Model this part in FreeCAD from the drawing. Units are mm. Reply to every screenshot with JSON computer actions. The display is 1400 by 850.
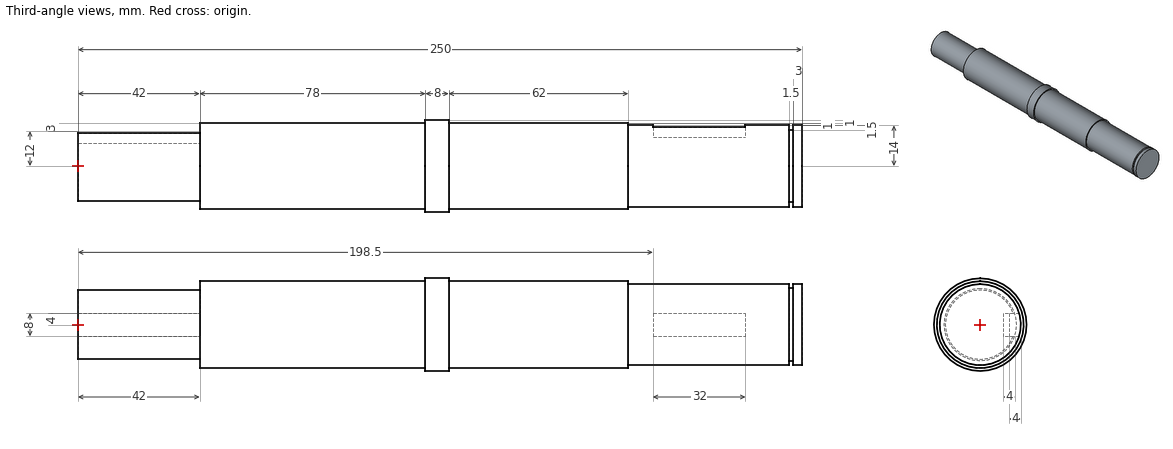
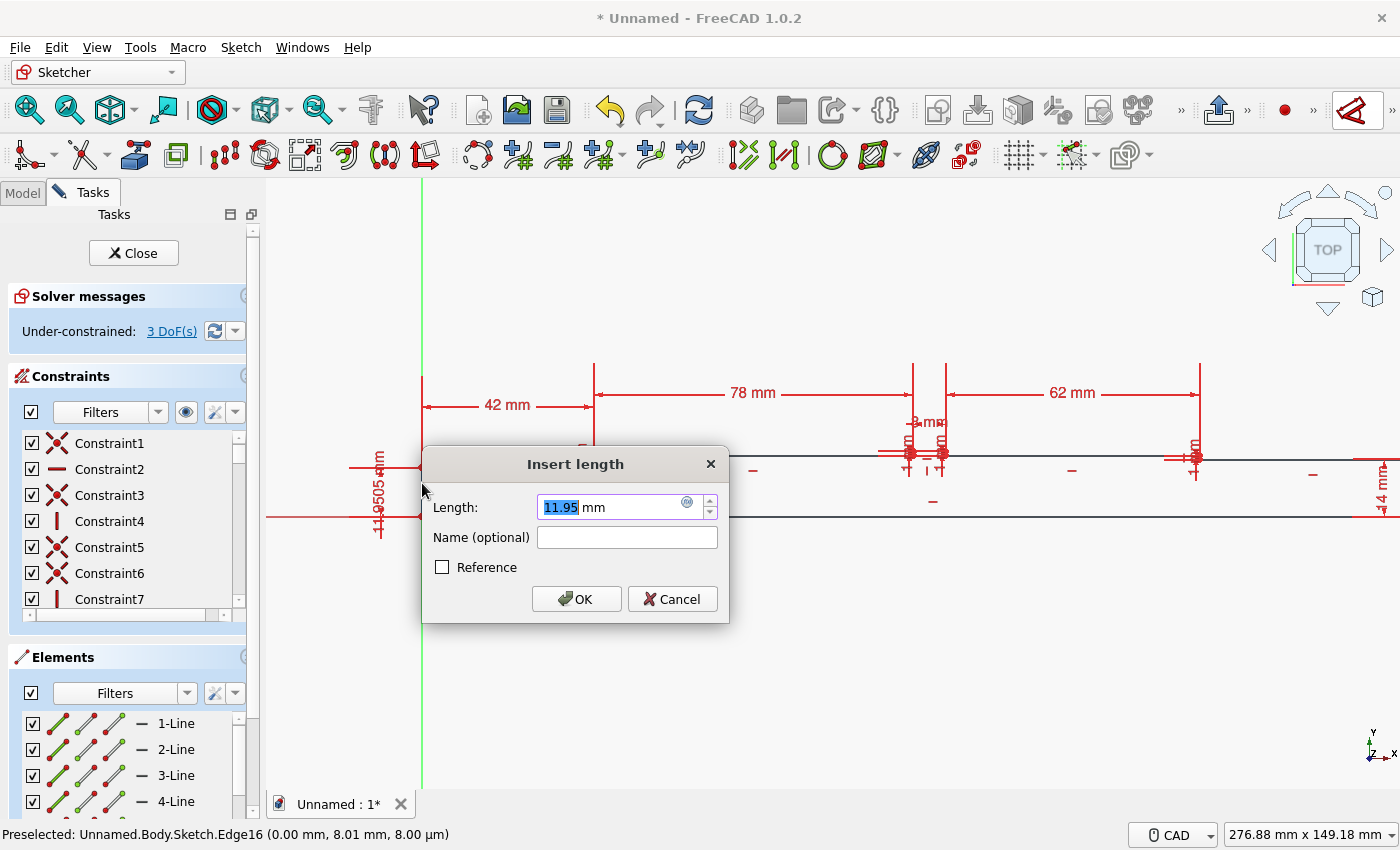
{"action": "type", "text": "12"}
{"action": "key", "text": "Return"}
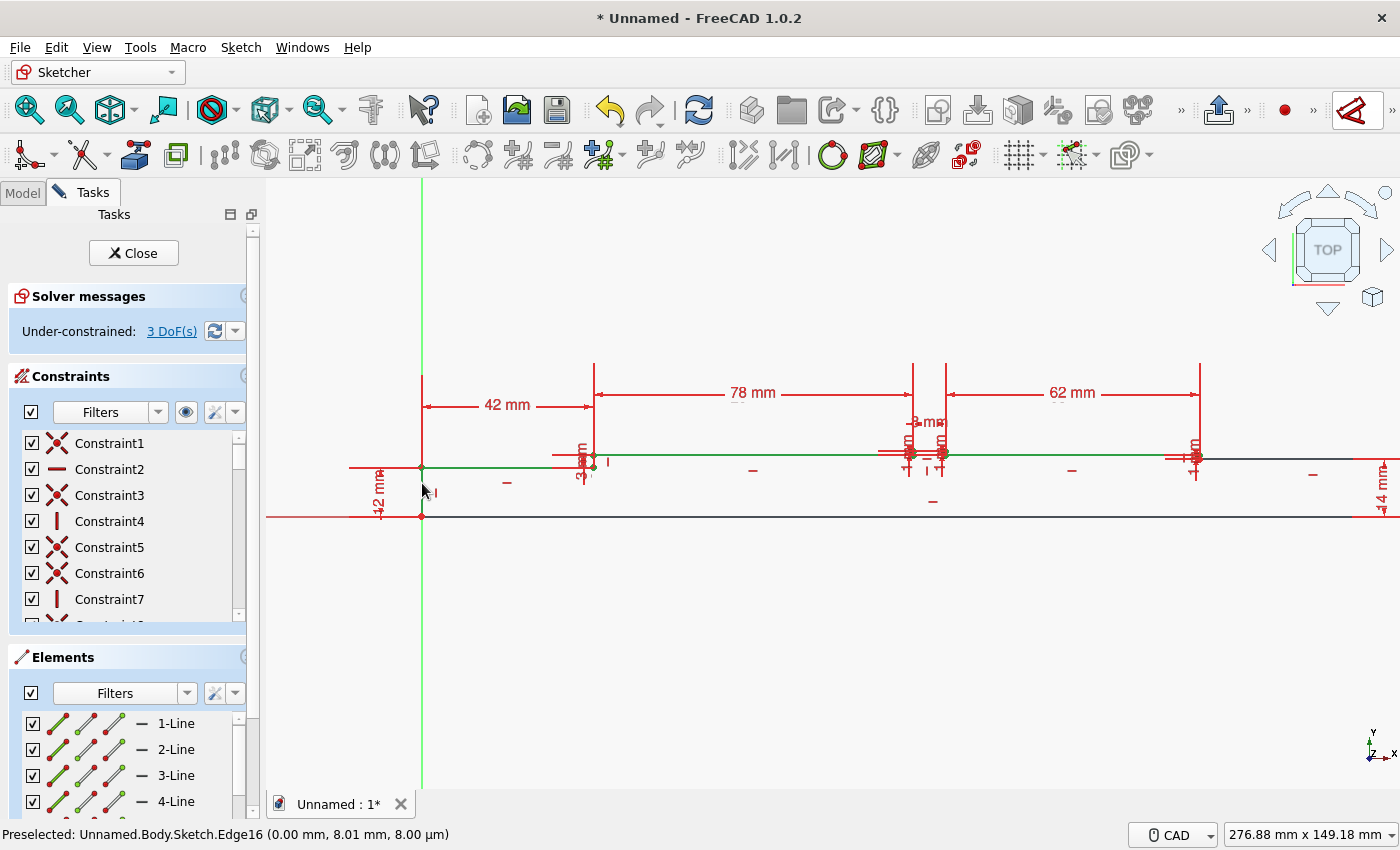
{"action": "left_click", "coordinate": [729, 517]}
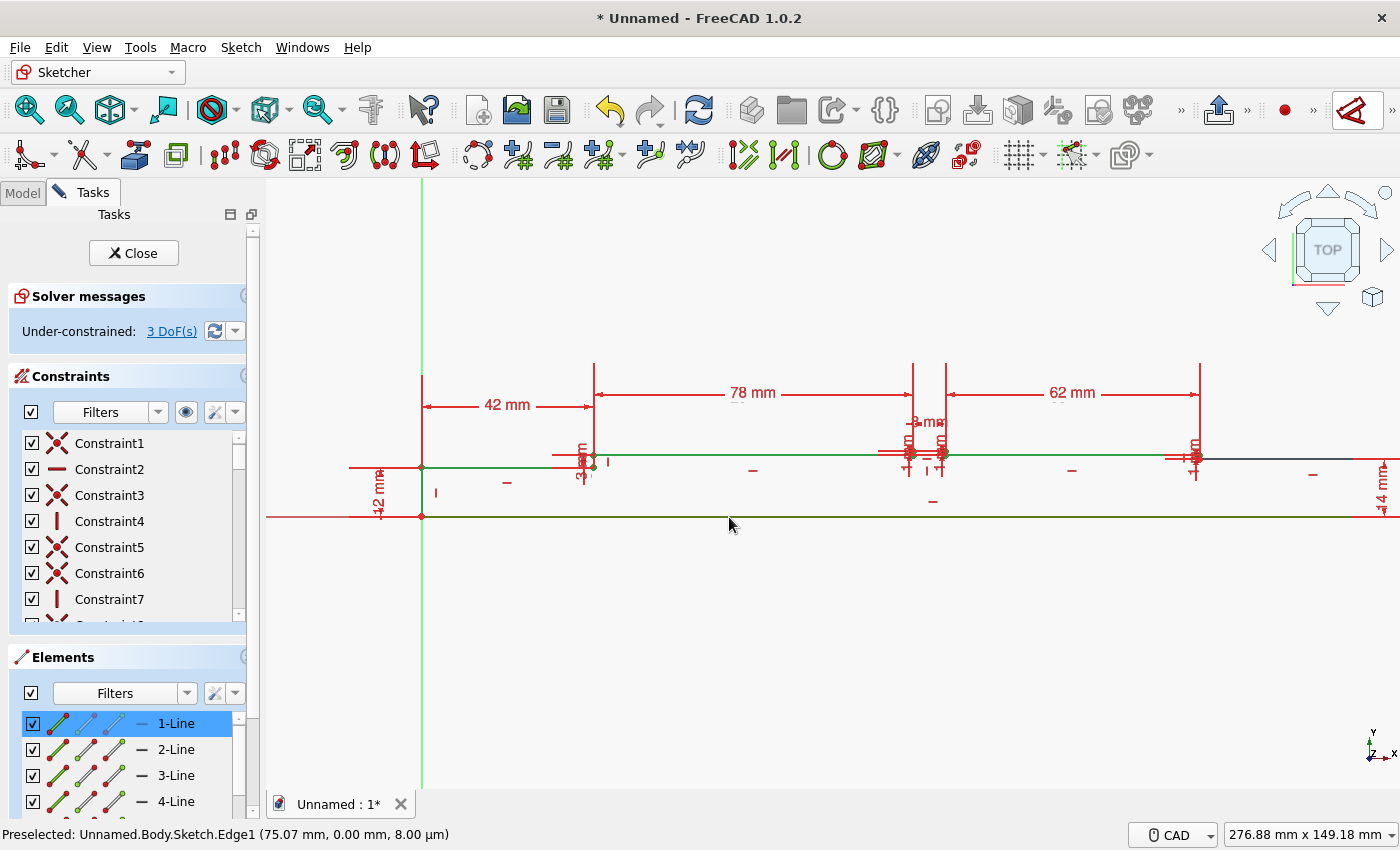
{"action": "left_click", "coordinate": [1378, 110]}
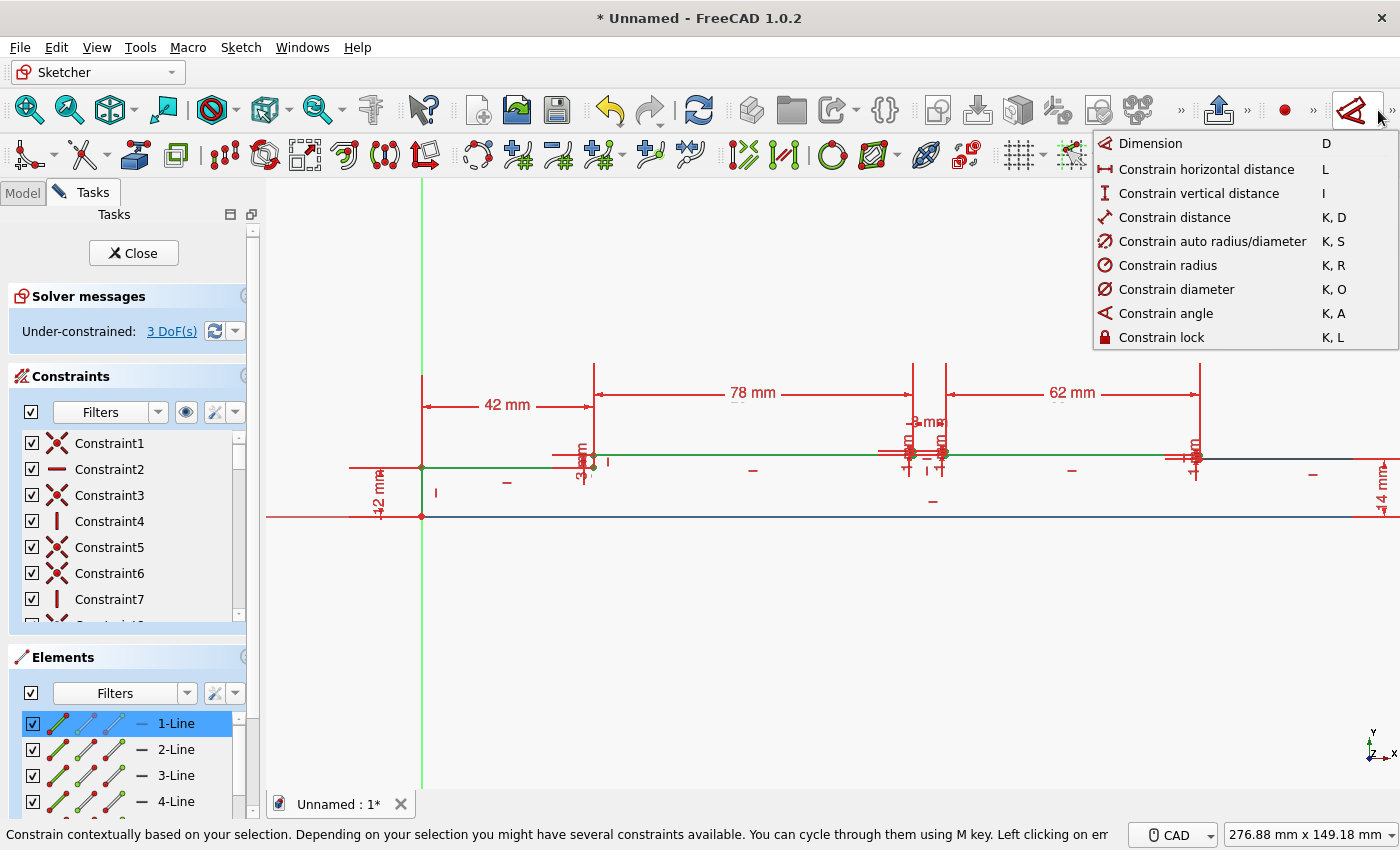
{"action": "left_click", "coordinate": [1246, 169]}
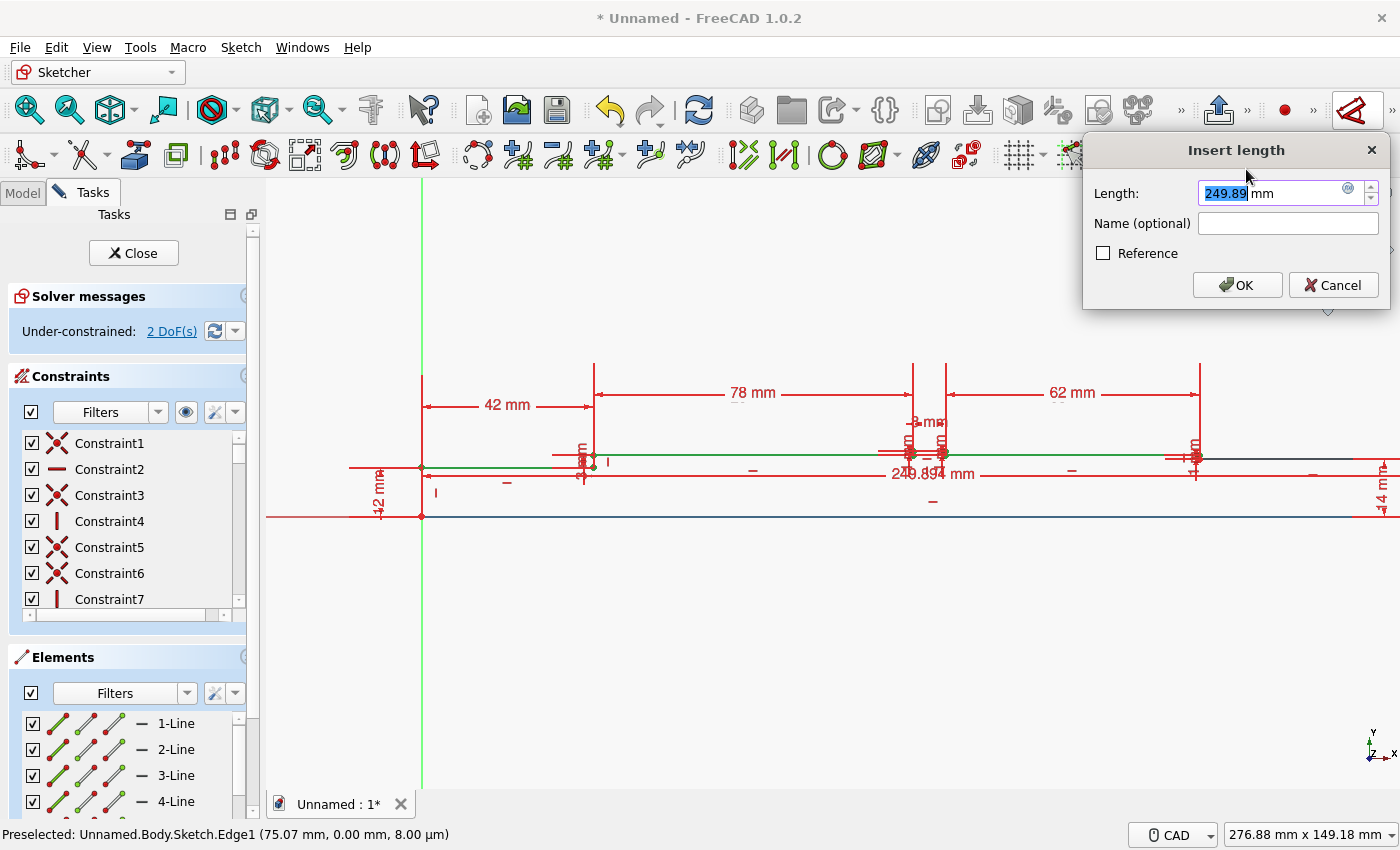
{"action": "type", "text": "250"}
{"action": "key", "text": "Return"}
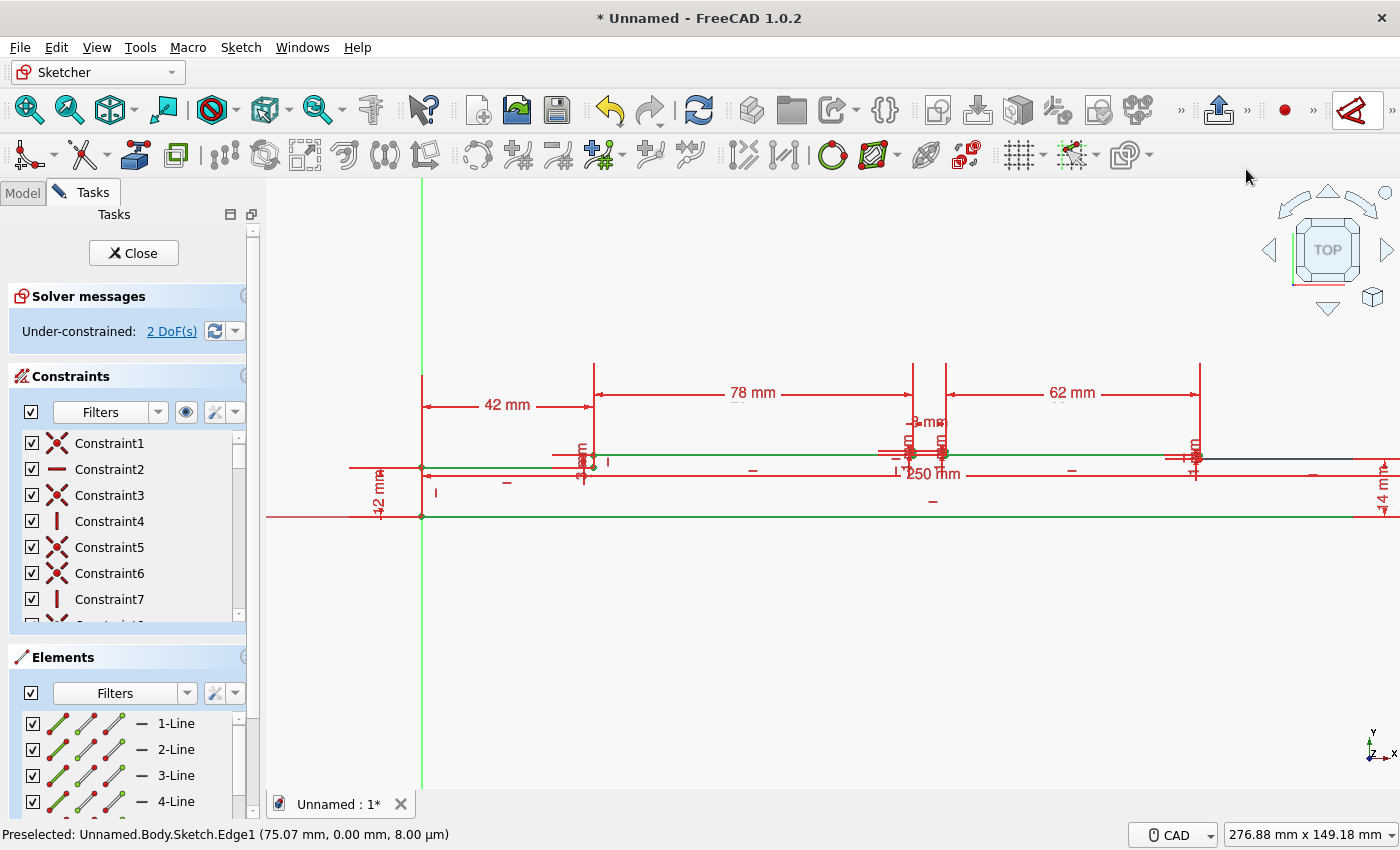
{"action": "scroll", "coordinate": [421, 482], "scroll_direction": "down", "scroll_amount": 2}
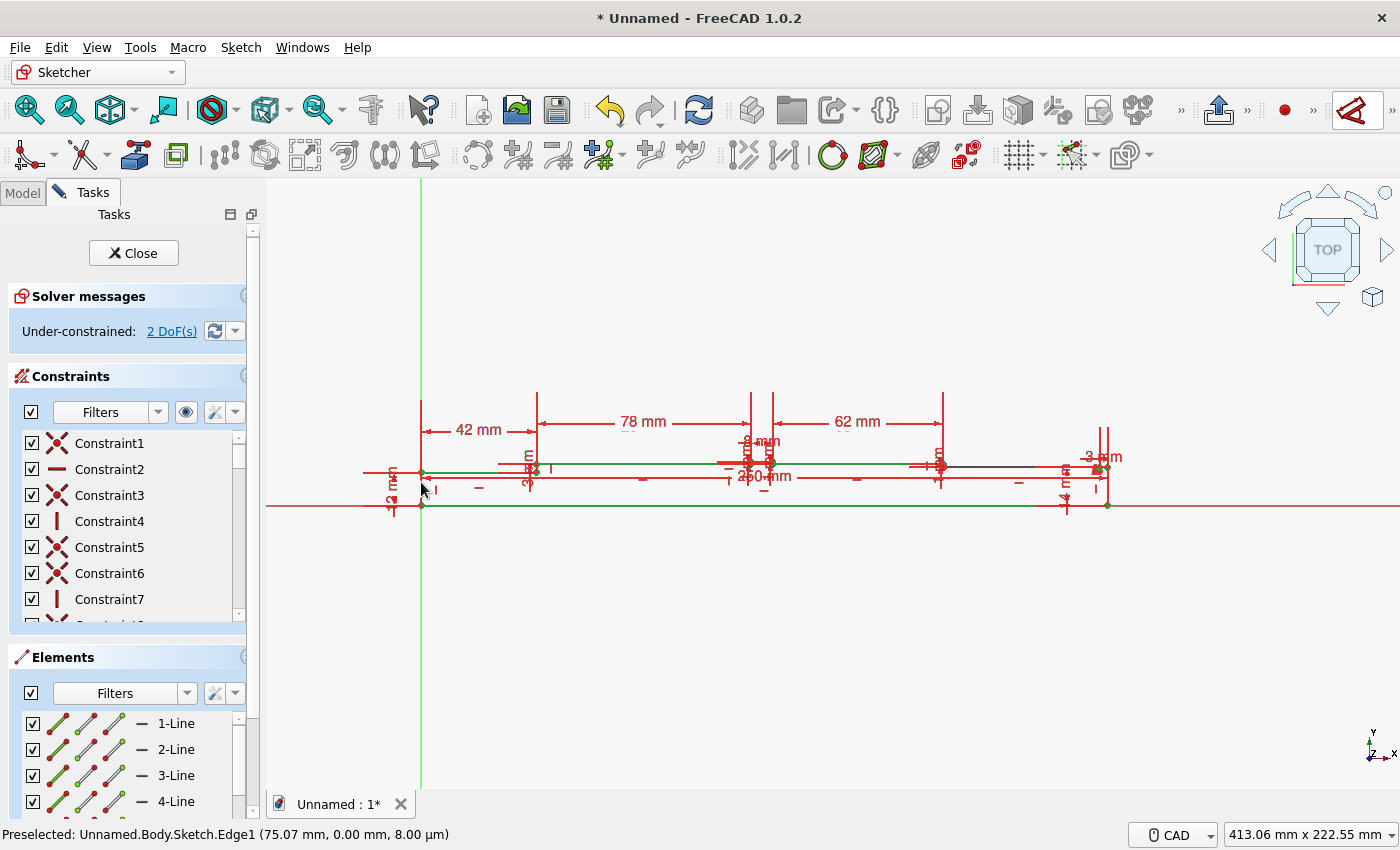
{"action": "scroll", "coordinate": [1100, 469], "scroll_direction": "up", "scroll_amount": 12}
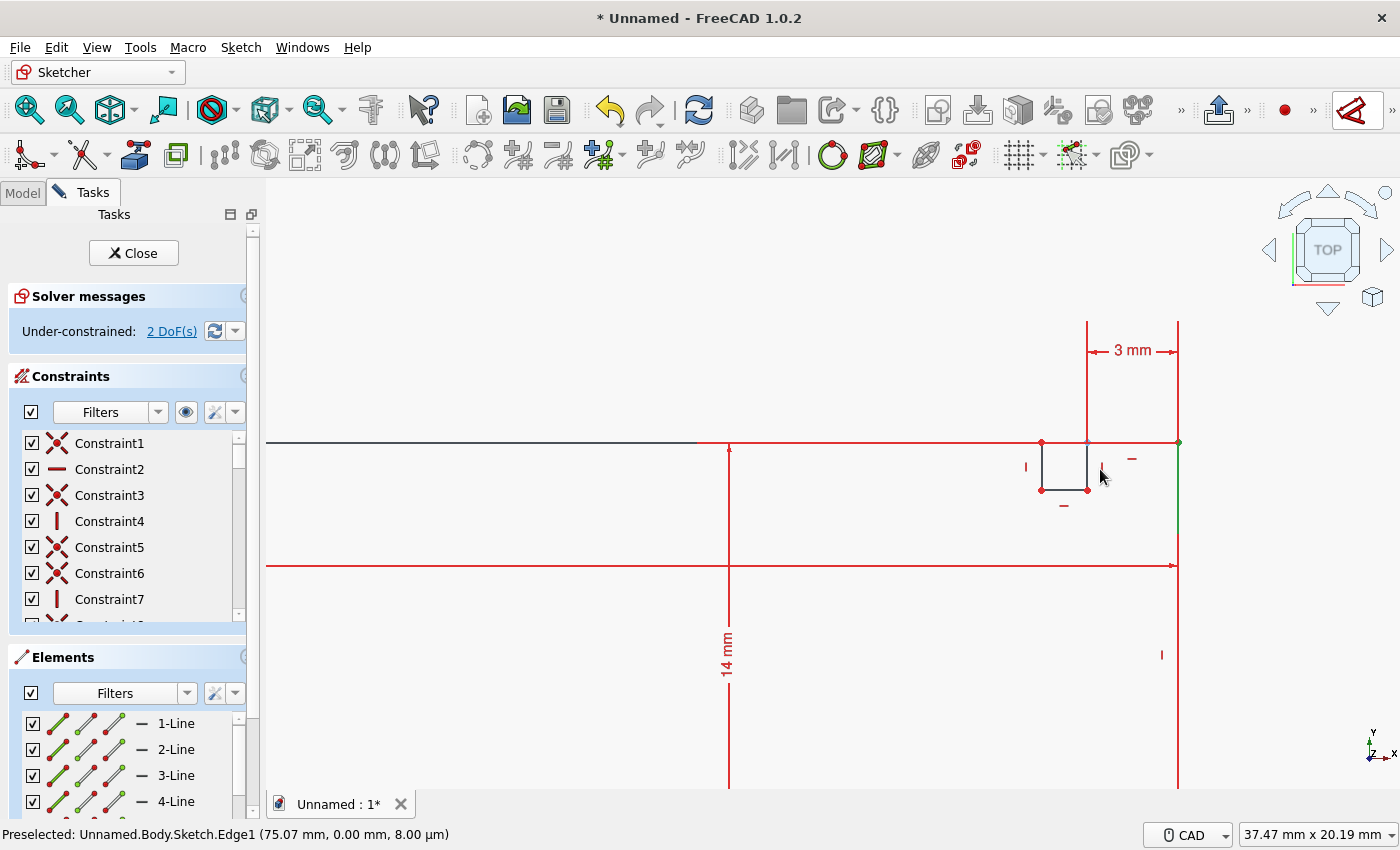
{"action": "left_click", "coordinate": [1087, 467]}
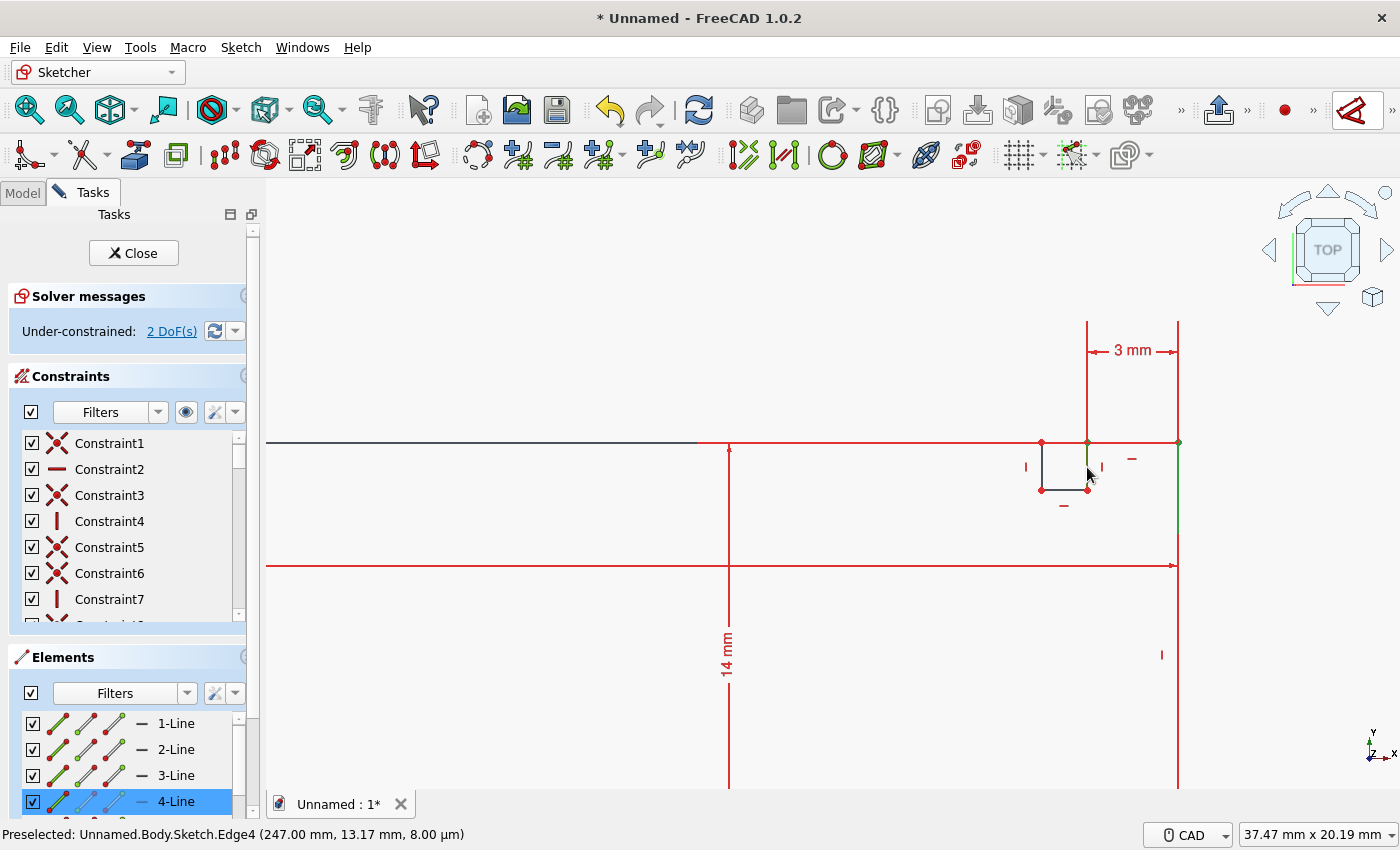
{"action": "key", "text": "i"}